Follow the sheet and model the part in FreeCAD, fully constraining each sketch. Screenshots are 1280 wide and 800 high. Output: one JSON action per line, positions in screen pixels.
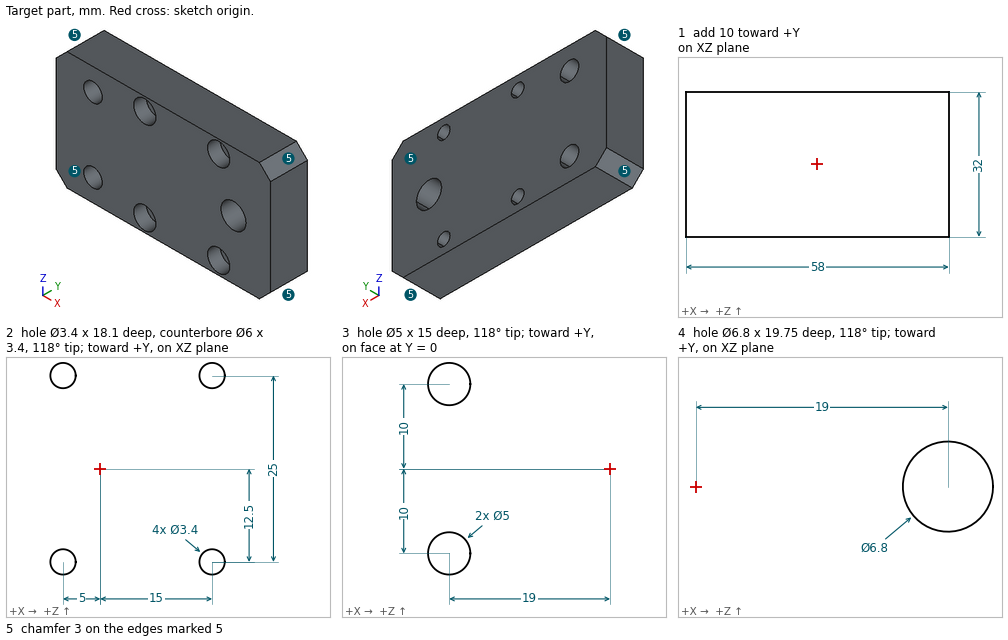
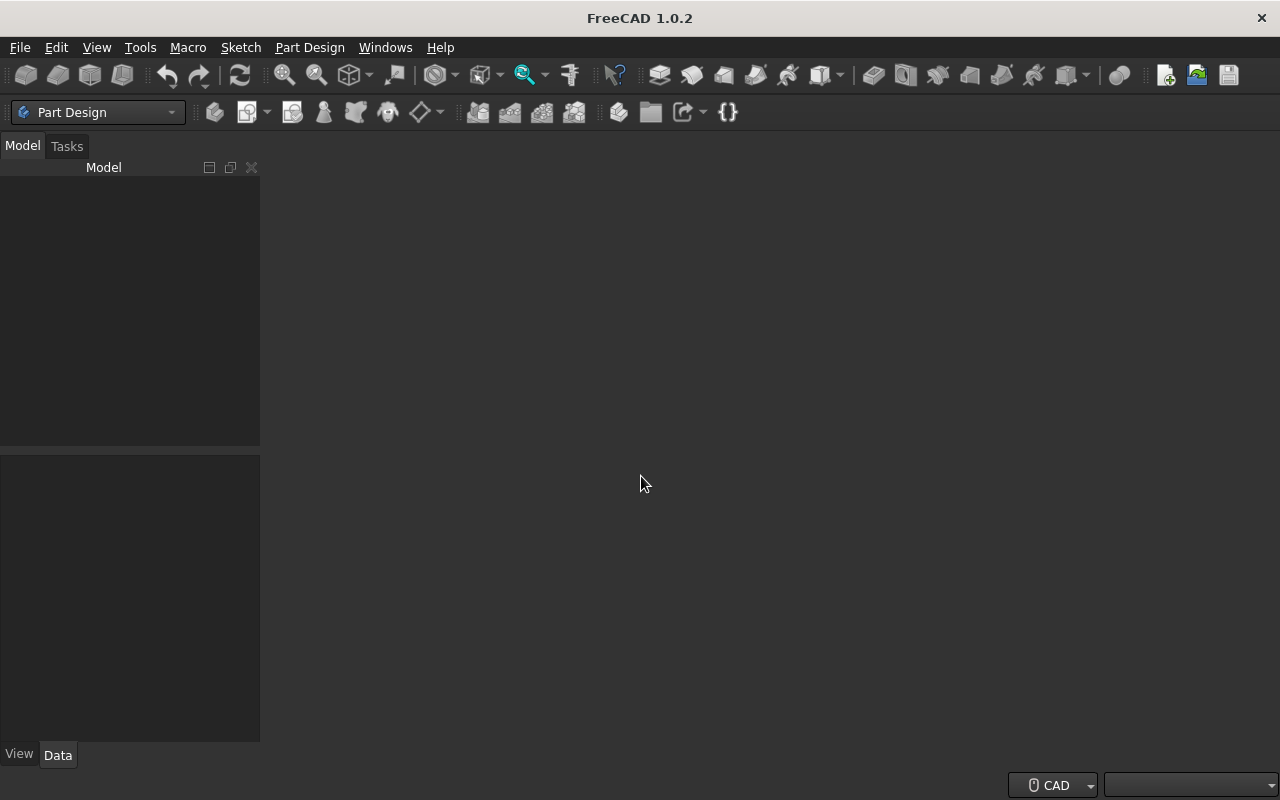
{"action": "left_click", "coordinate": [1166, 76]}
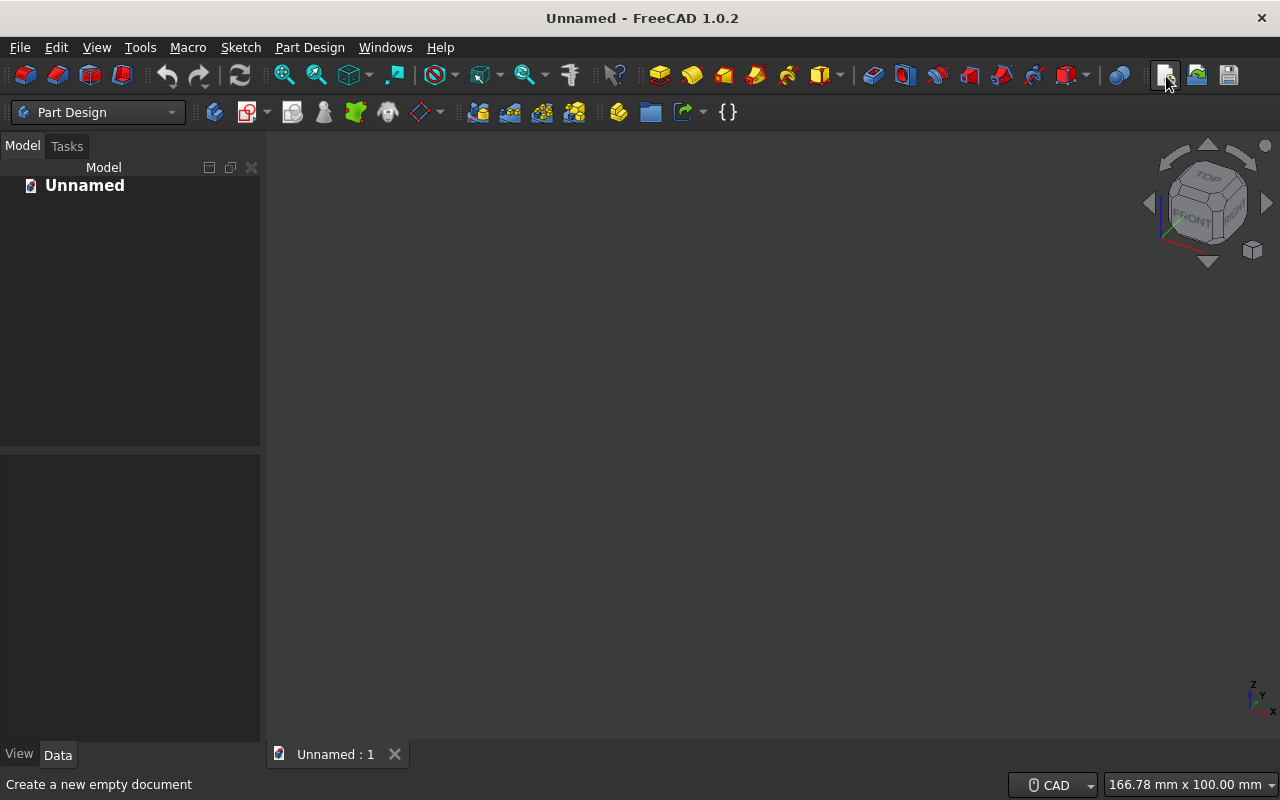
{"action": "left_click", "coordinate": [248, 112]}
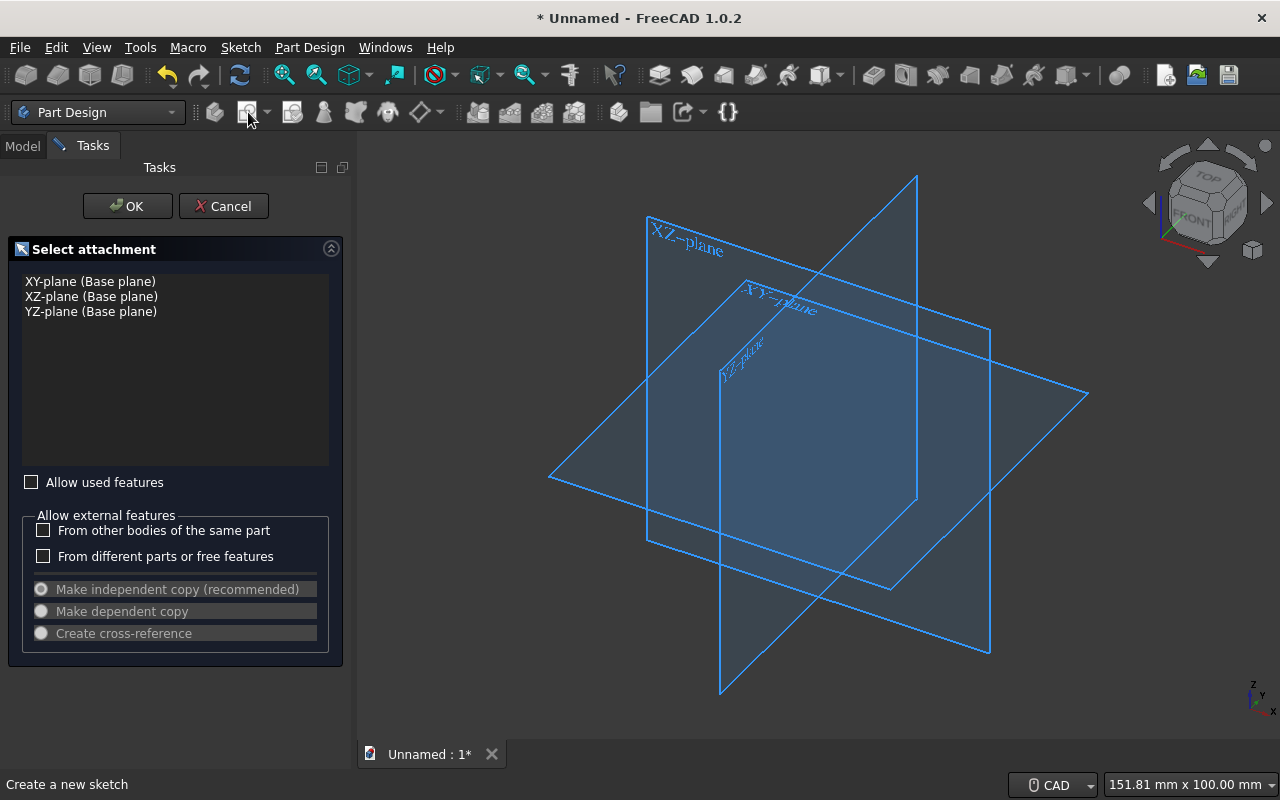
{"action": "left_click", "coordinate": [82, 296]}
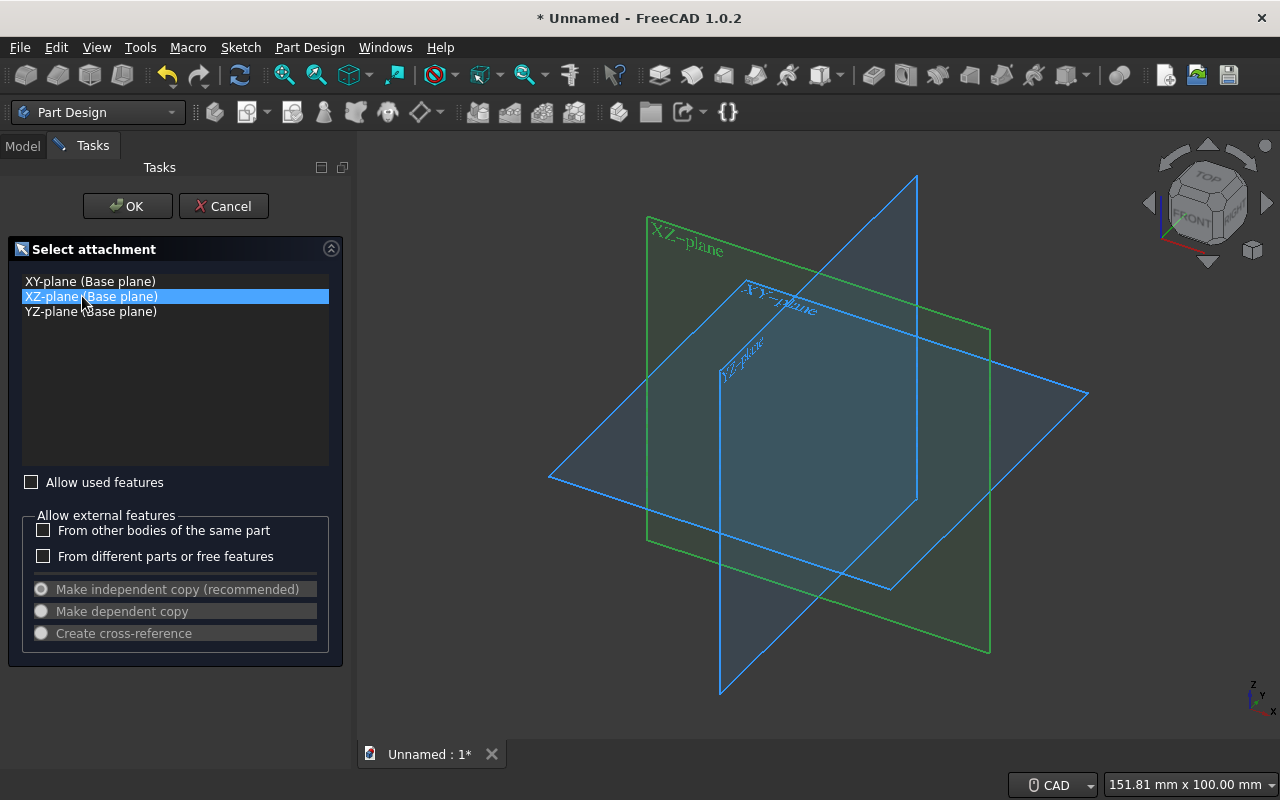
{"action": "left_click", "coordinate": [128, 206]}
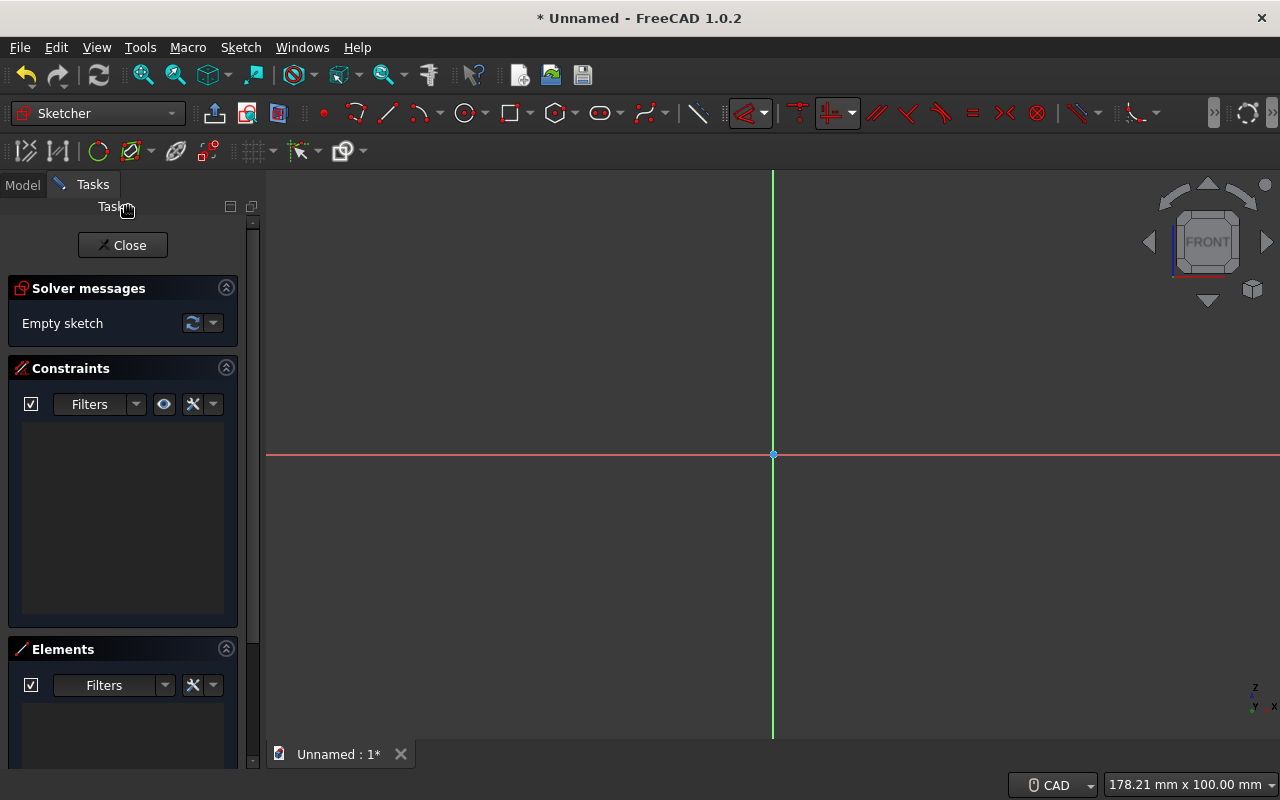
{"action": "scroll", "coordinate": [856, 454], "scroll_direction": "up", "scroll_amount": 3}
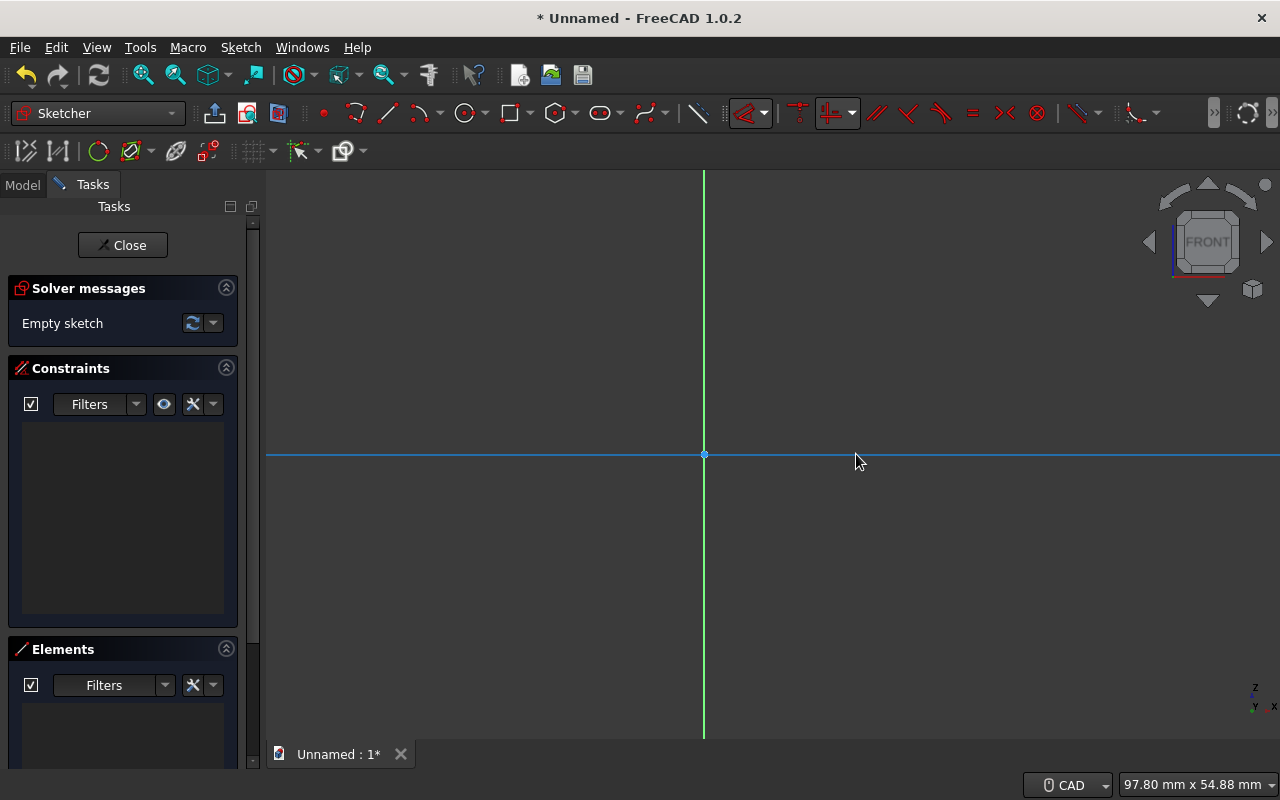
{"action": "left_click", "coordinate": [532, 114]}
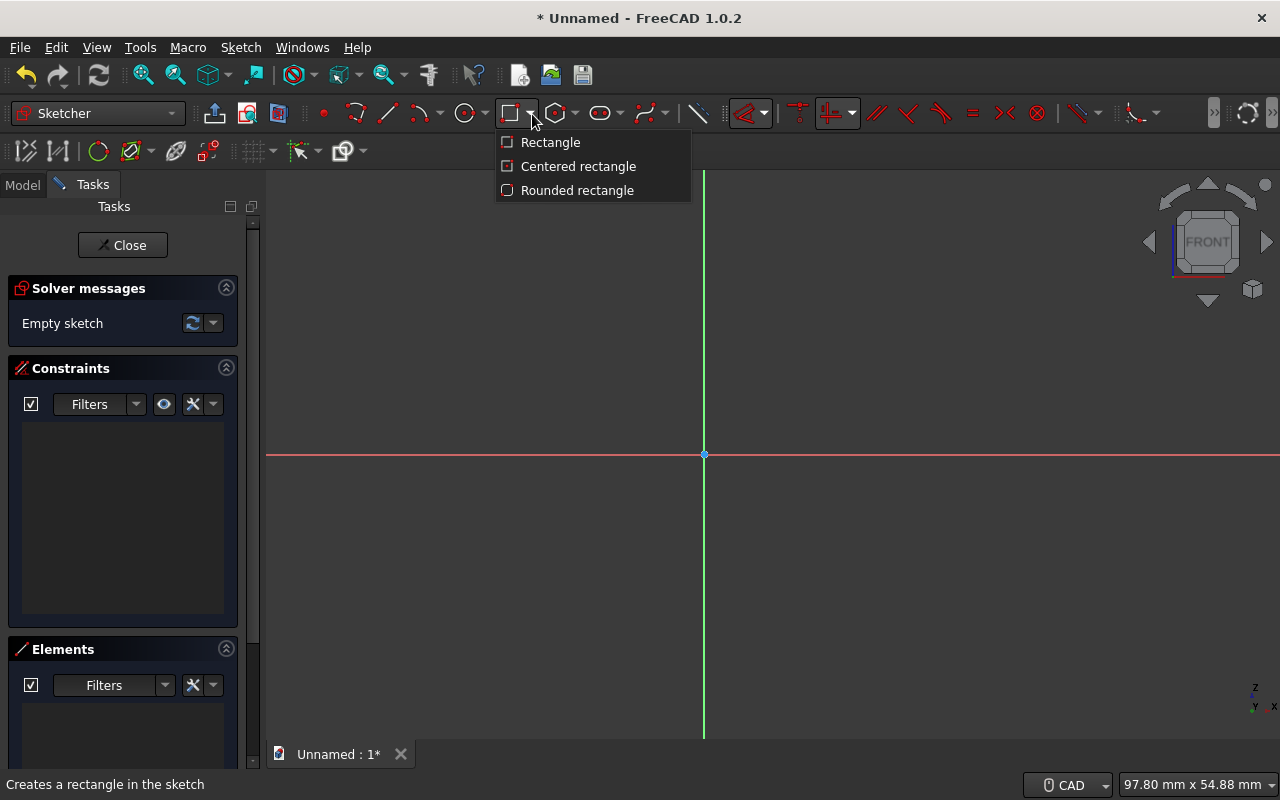
{"action": "left_click", "coordinate": [594, 166]}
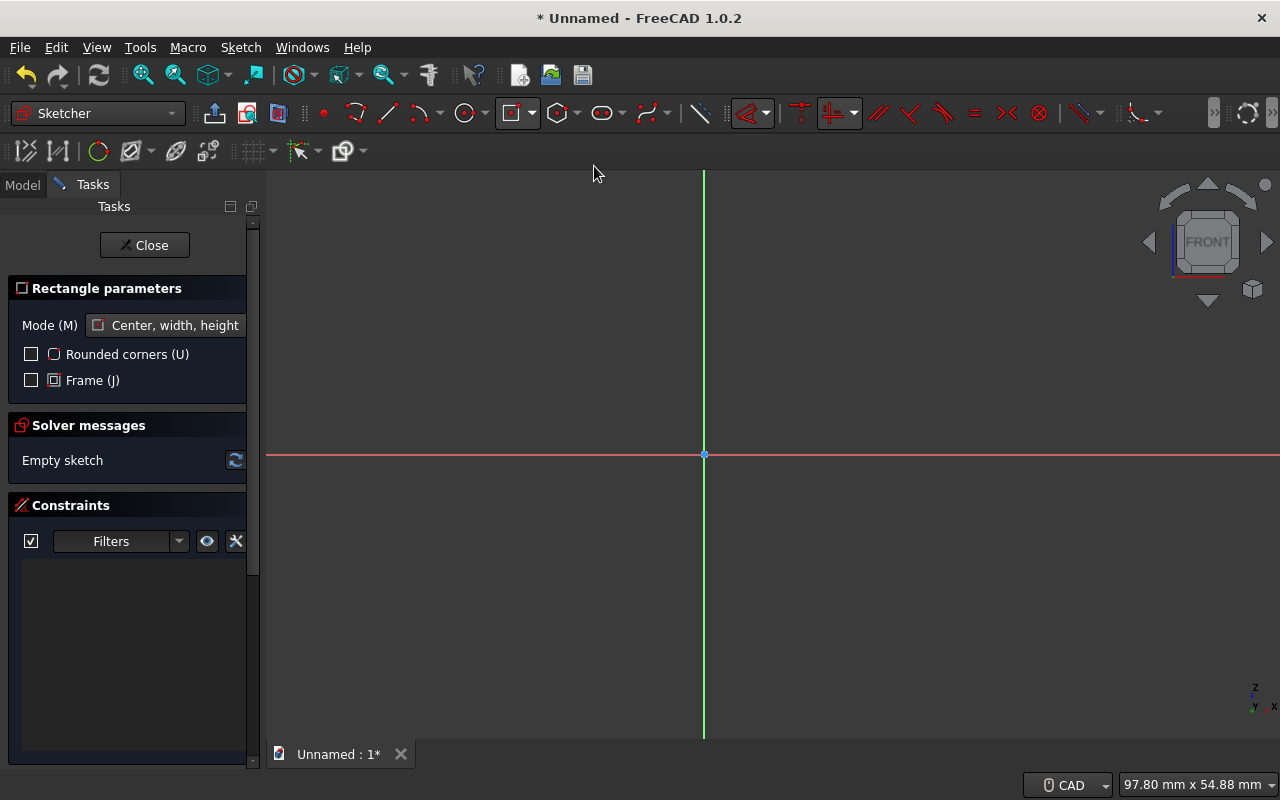
{"action": "left_click", "coordinate": [704, 454]}
{"action": "left_click", "coordinate": [1005, 289]}
{"action": "key", "text": "Escape"}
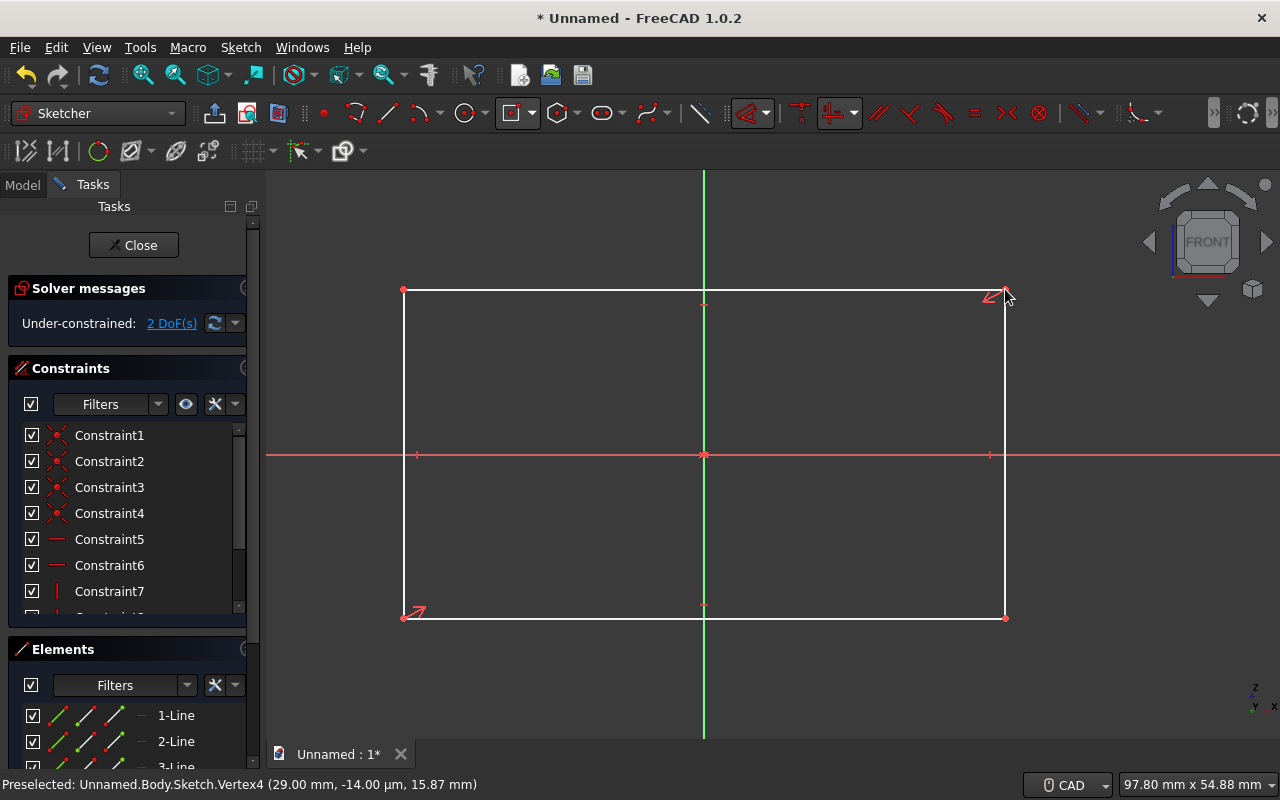
{"action": "left_click", "coordinate": [746, 114]}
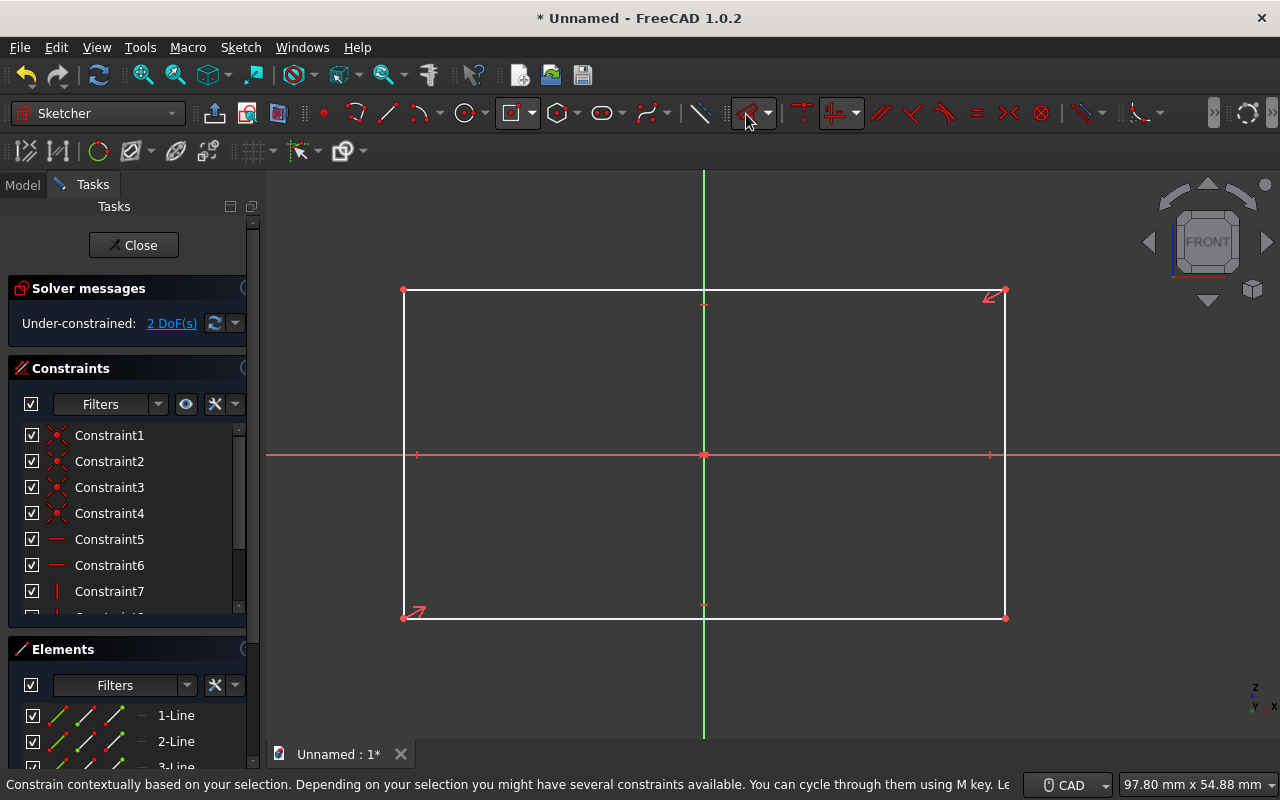
{"action": "left_click", "coordinate": [584, 619]}
{"action": "left_click", "coordinate": [566, 653]}